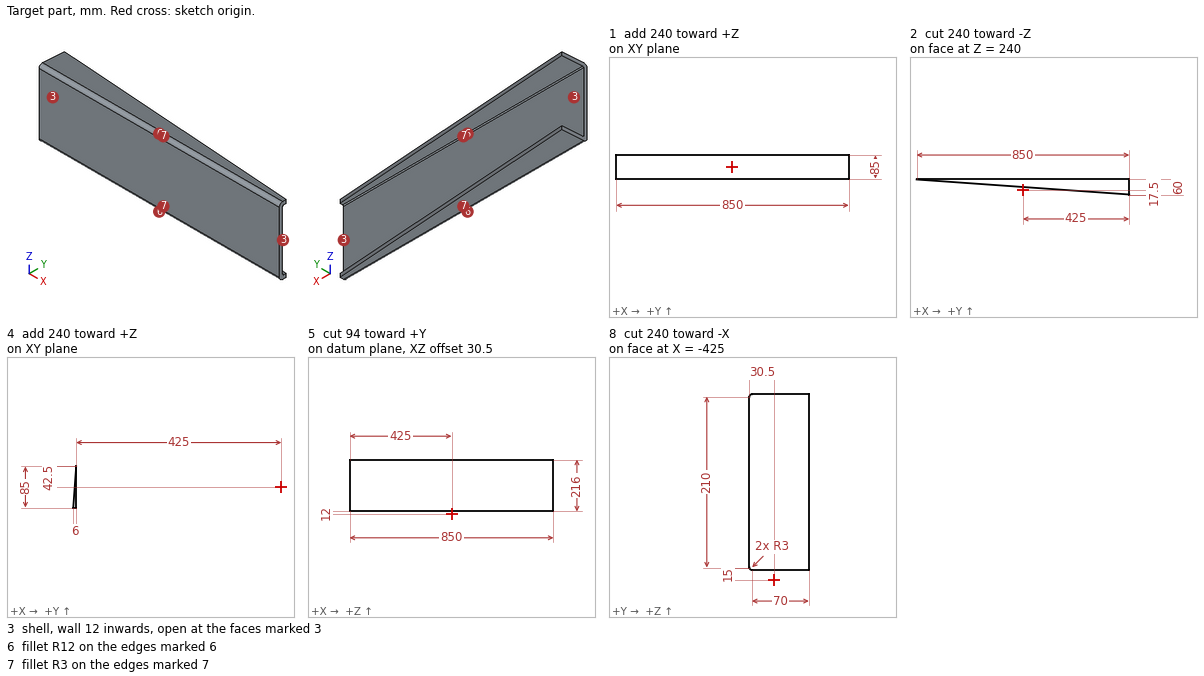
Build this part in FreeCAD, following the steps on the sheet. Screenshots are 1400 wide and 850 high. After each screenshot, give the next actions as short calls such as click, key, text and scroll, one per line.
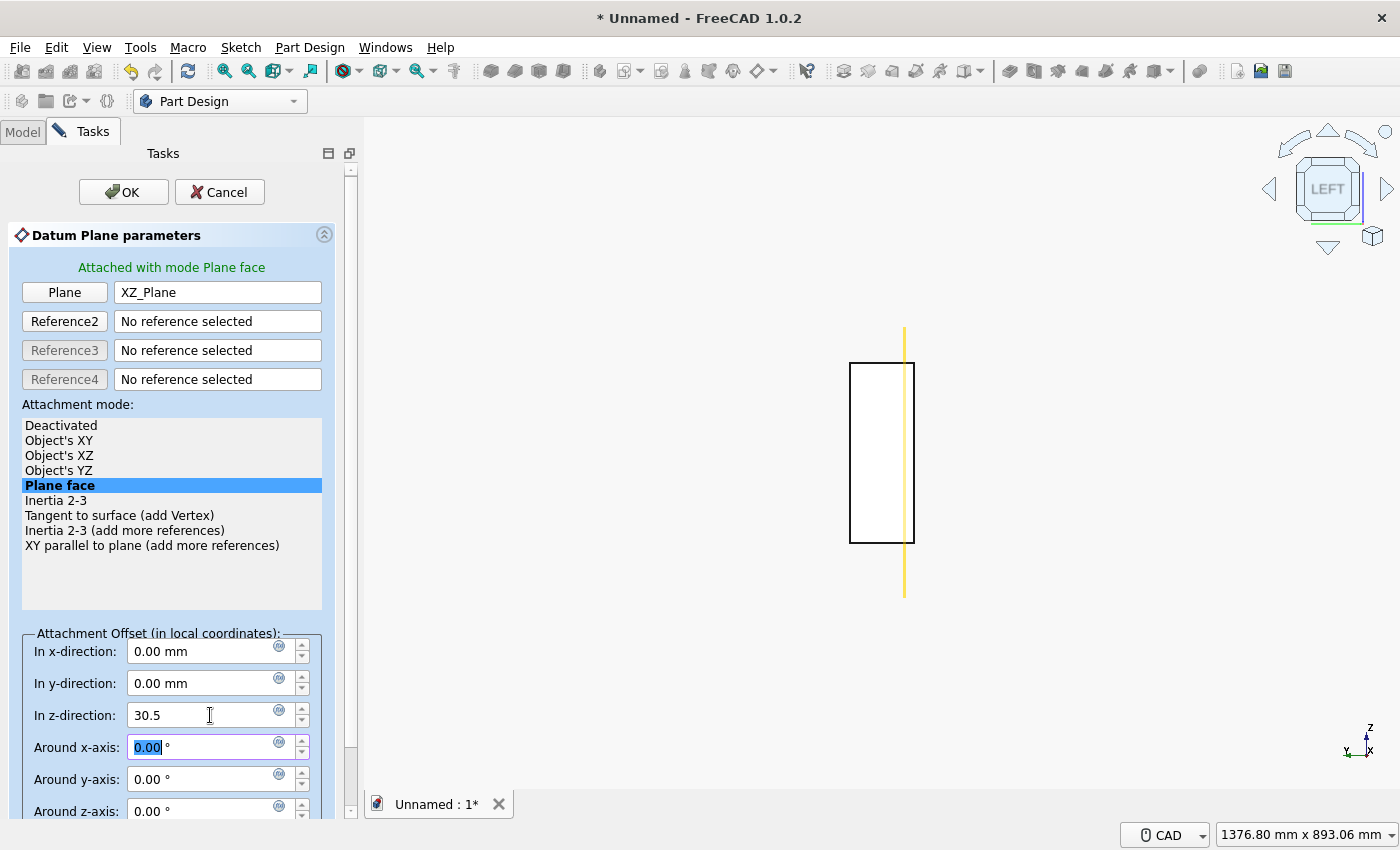
click(124, 192)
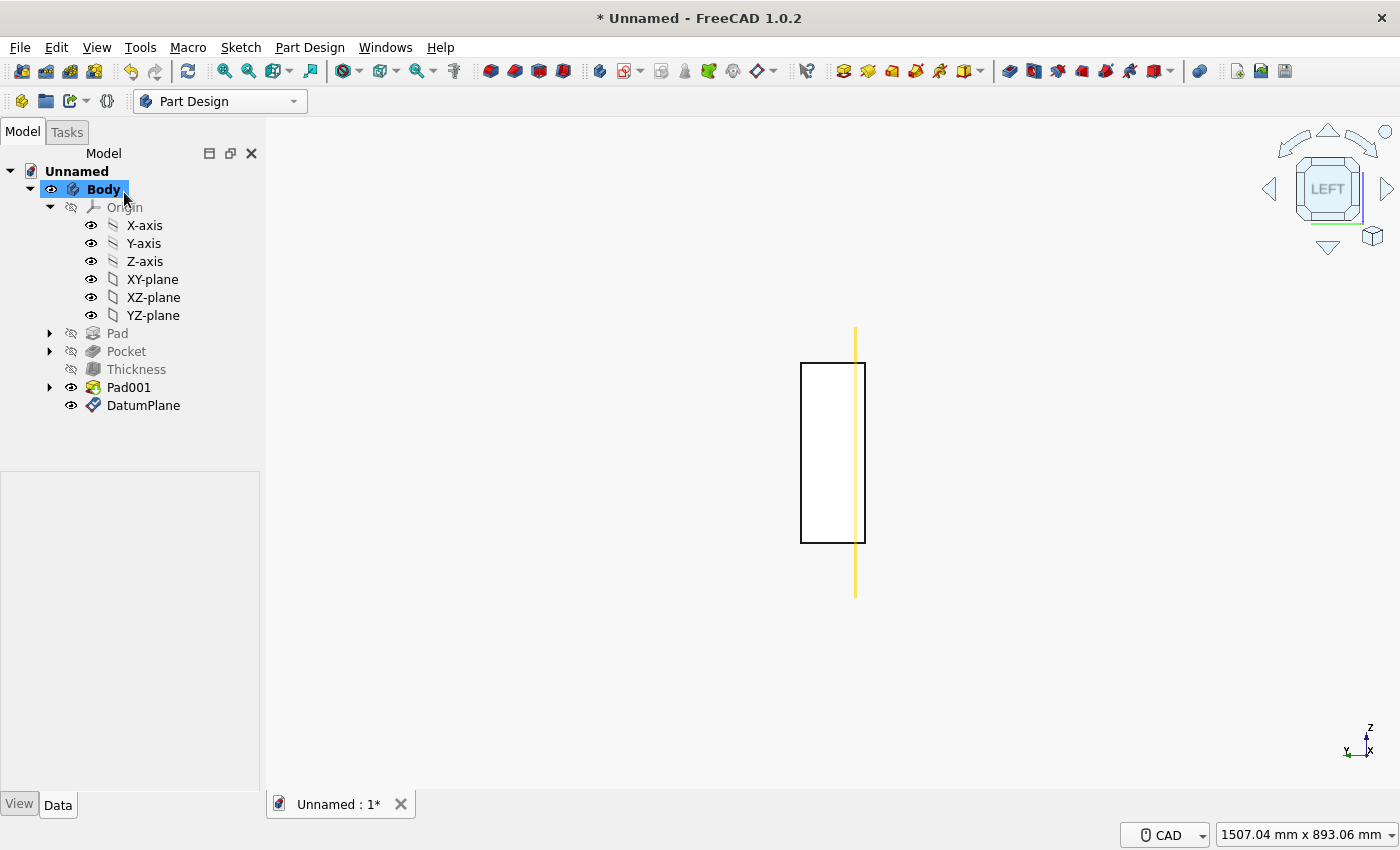
click(116, 405)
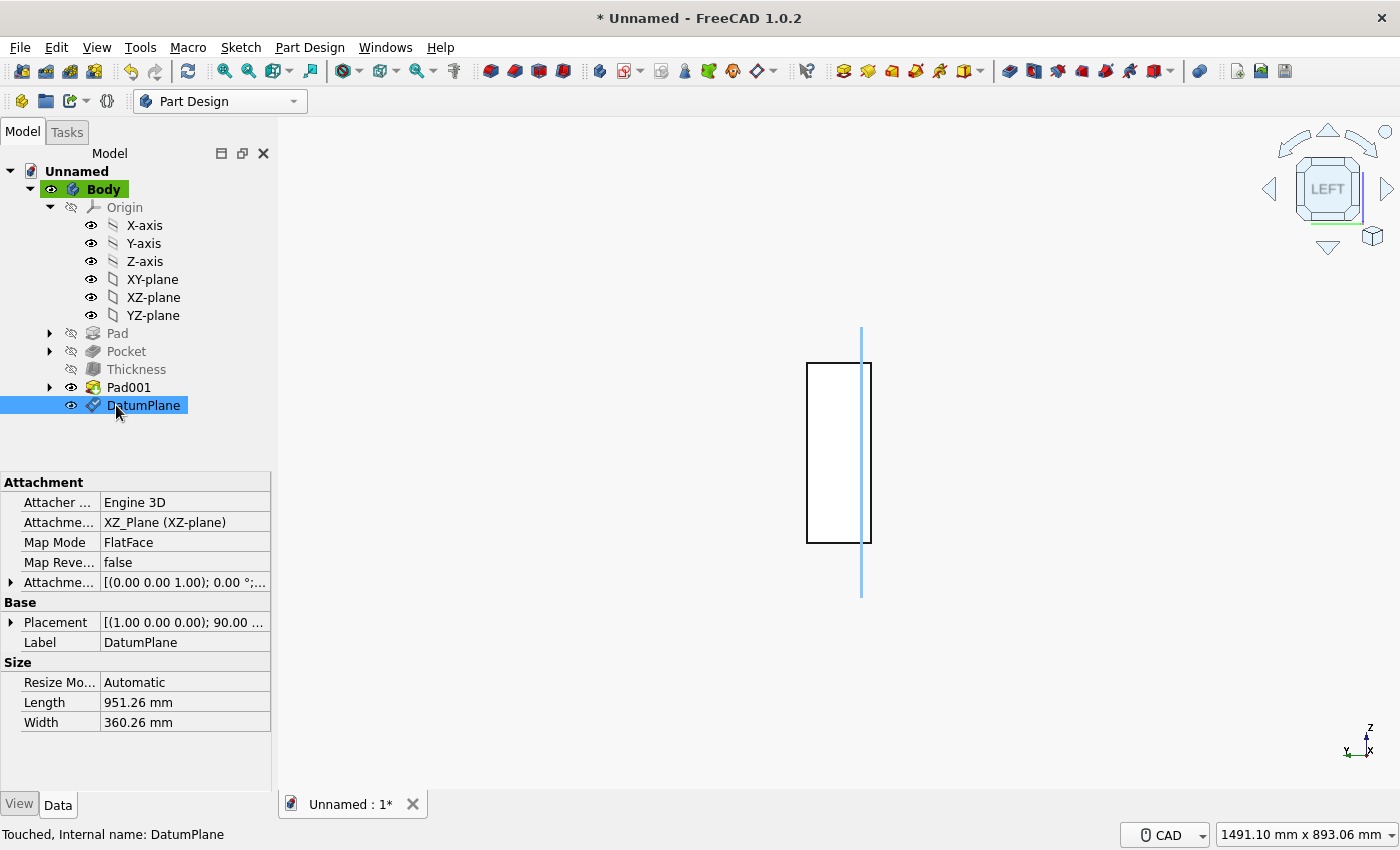
click(624, 72)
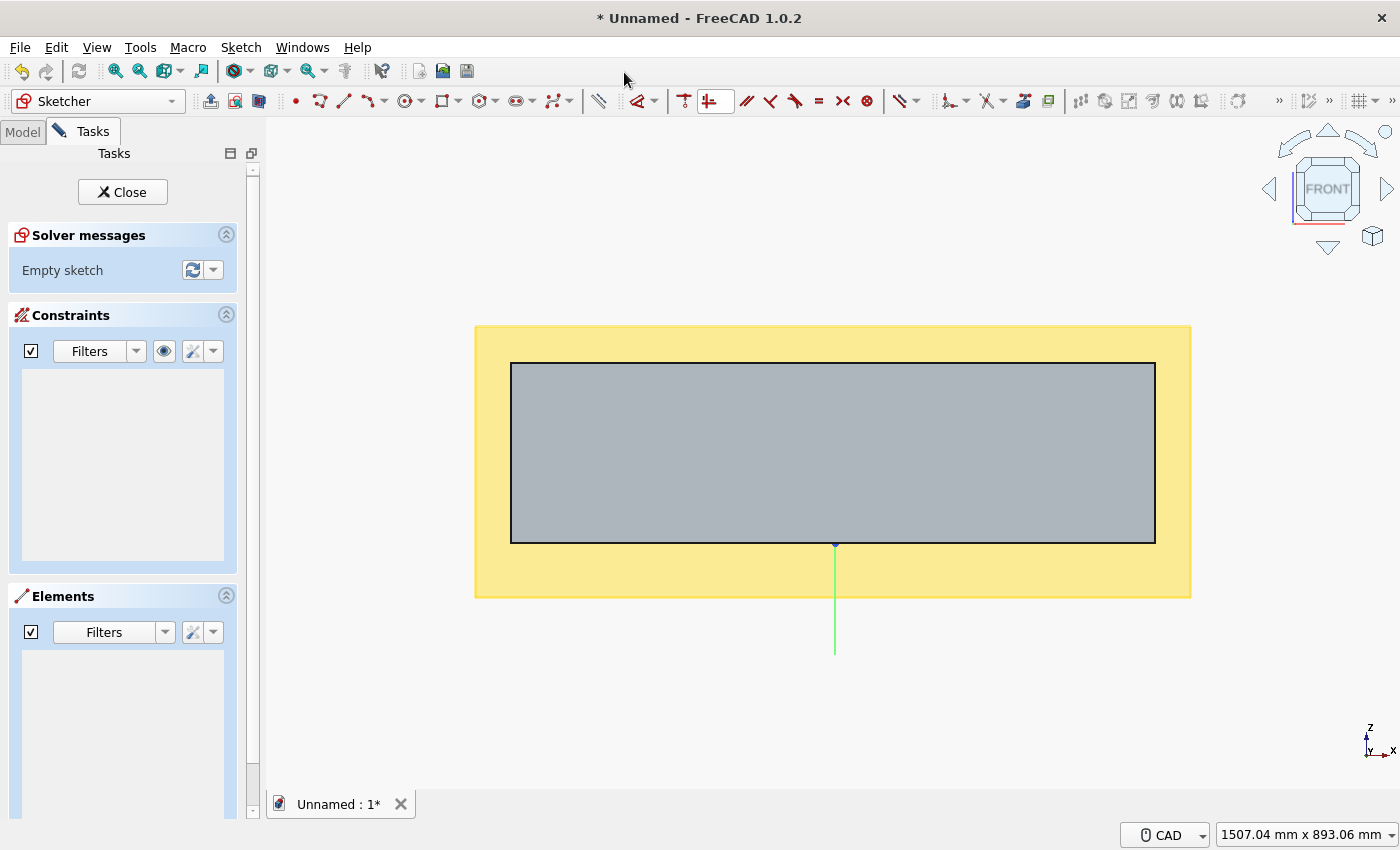
key(q)
key(s)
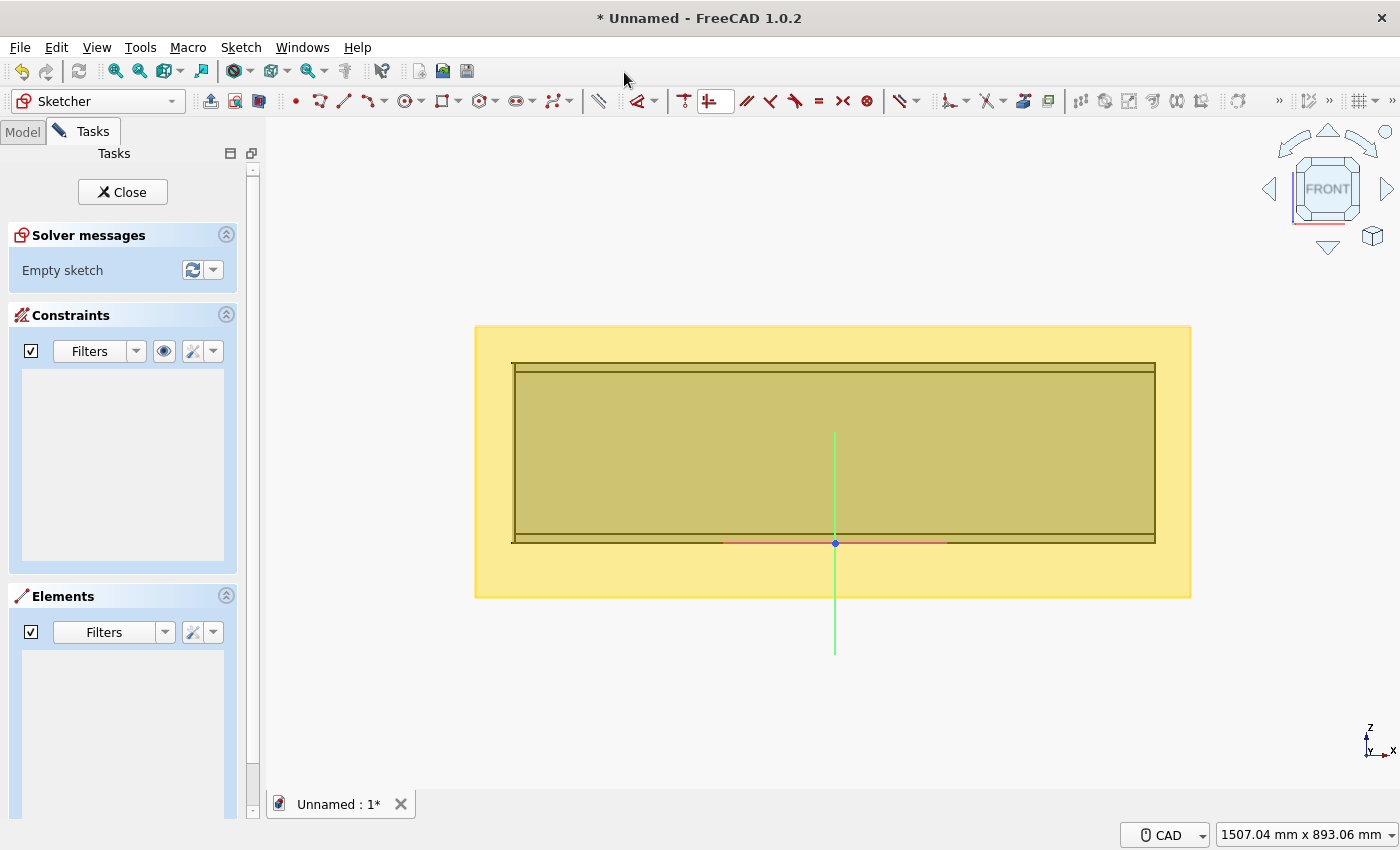
click(442, 102)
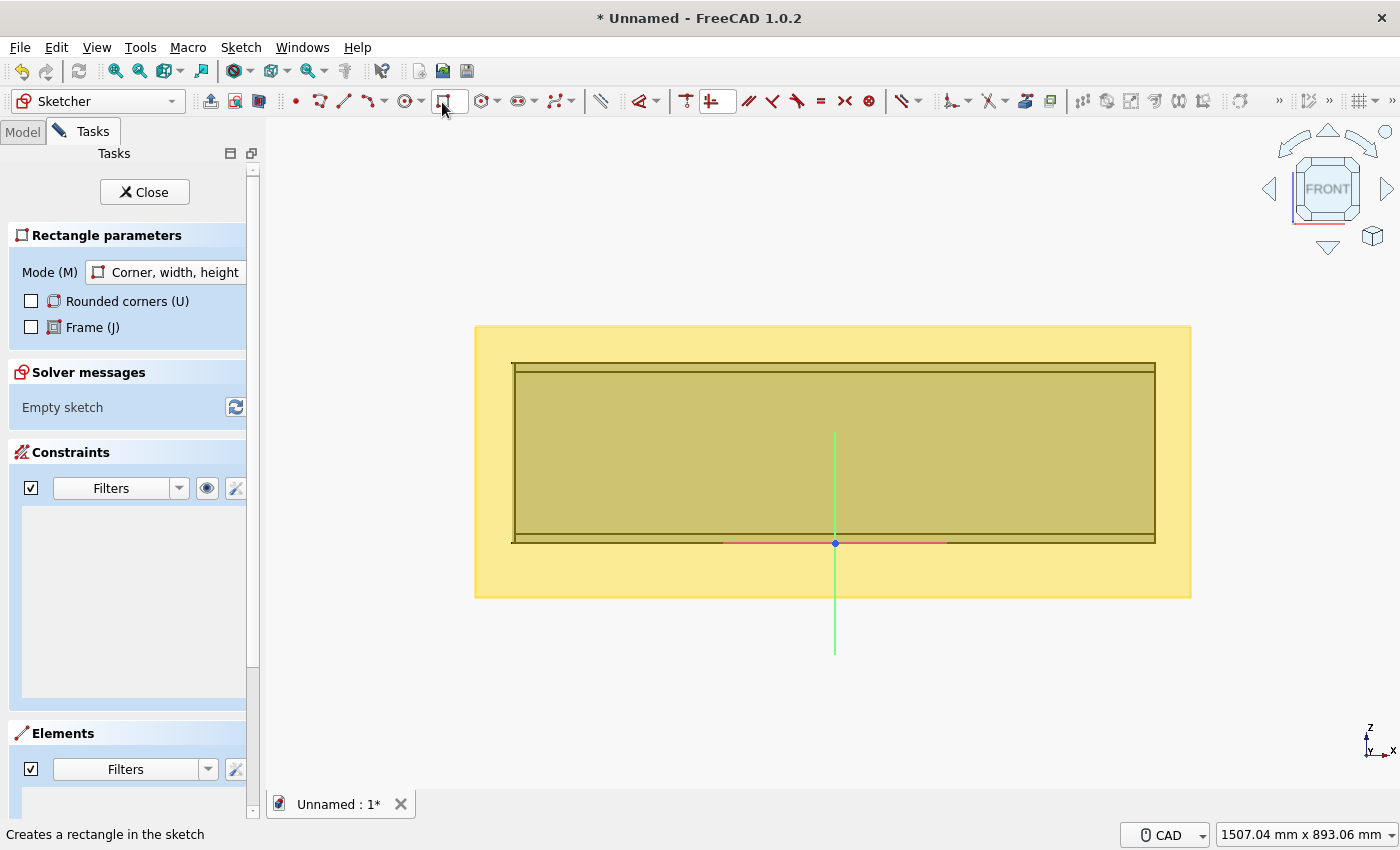
click(515, 372)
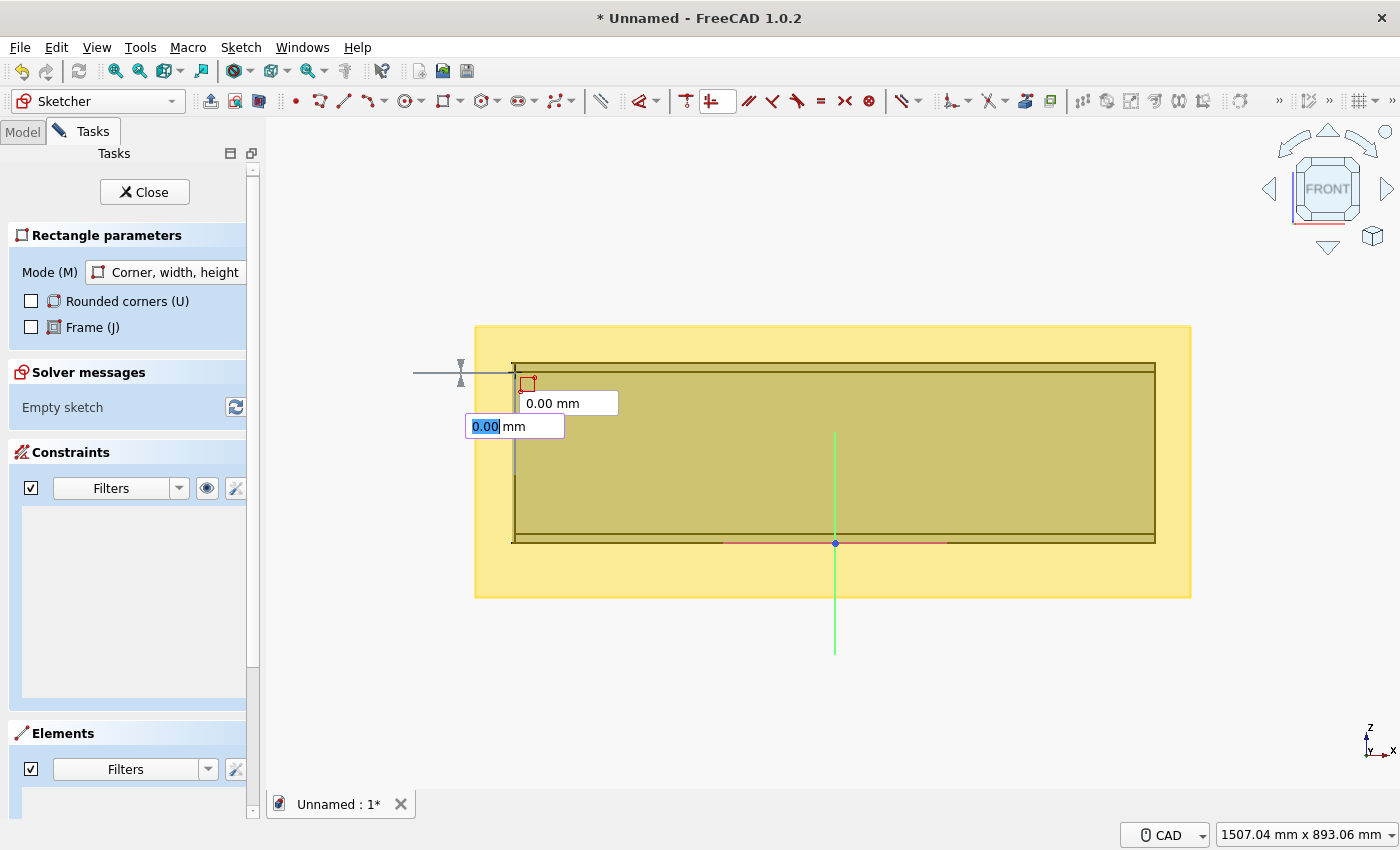
scroll(1155, 534, up, 3)
move(1154, 534)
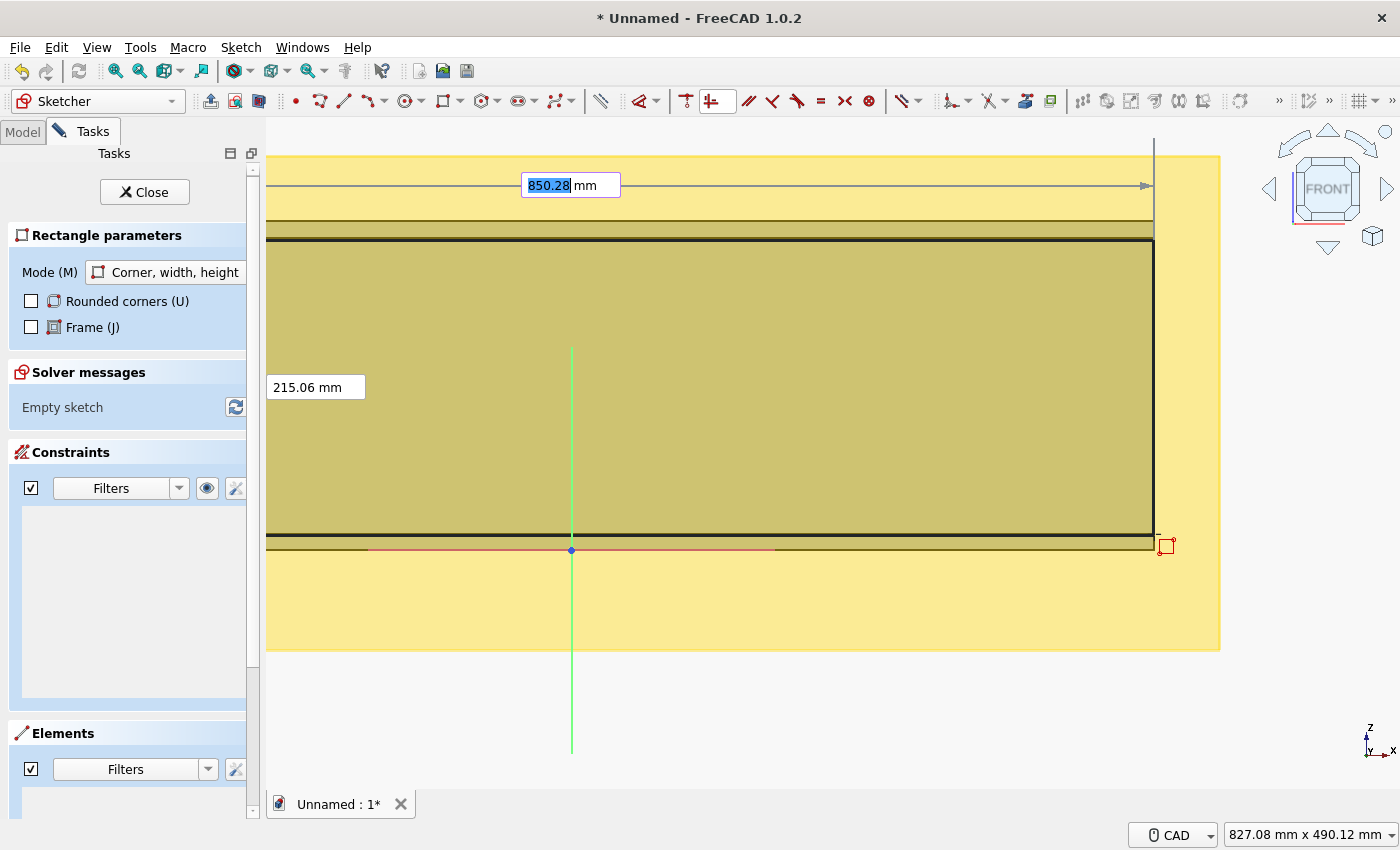
text(850)
key(Tab)
text(216)
key(Return)
key(Escape)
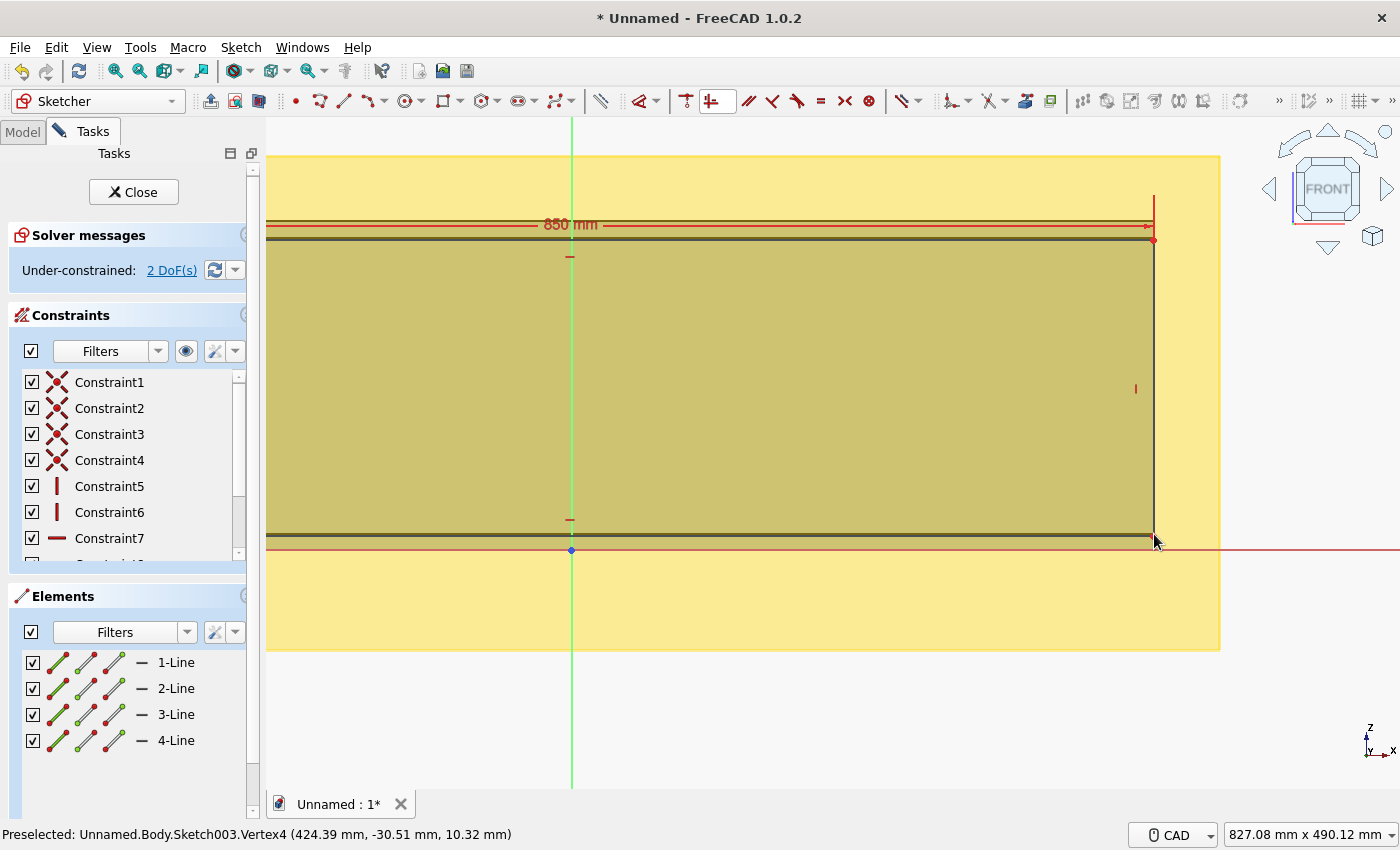
key(d)